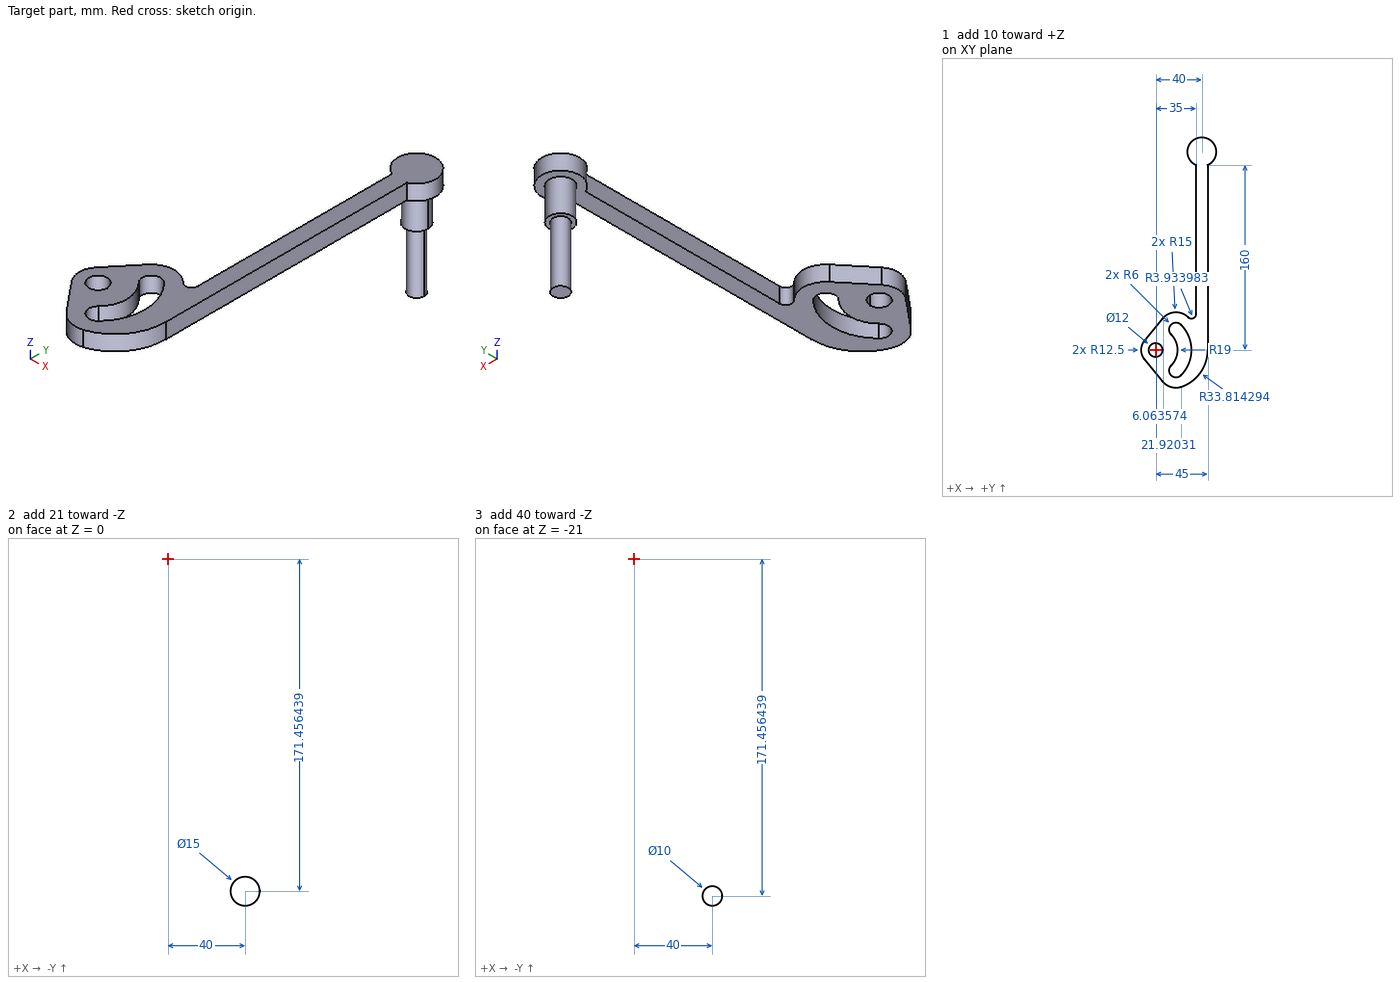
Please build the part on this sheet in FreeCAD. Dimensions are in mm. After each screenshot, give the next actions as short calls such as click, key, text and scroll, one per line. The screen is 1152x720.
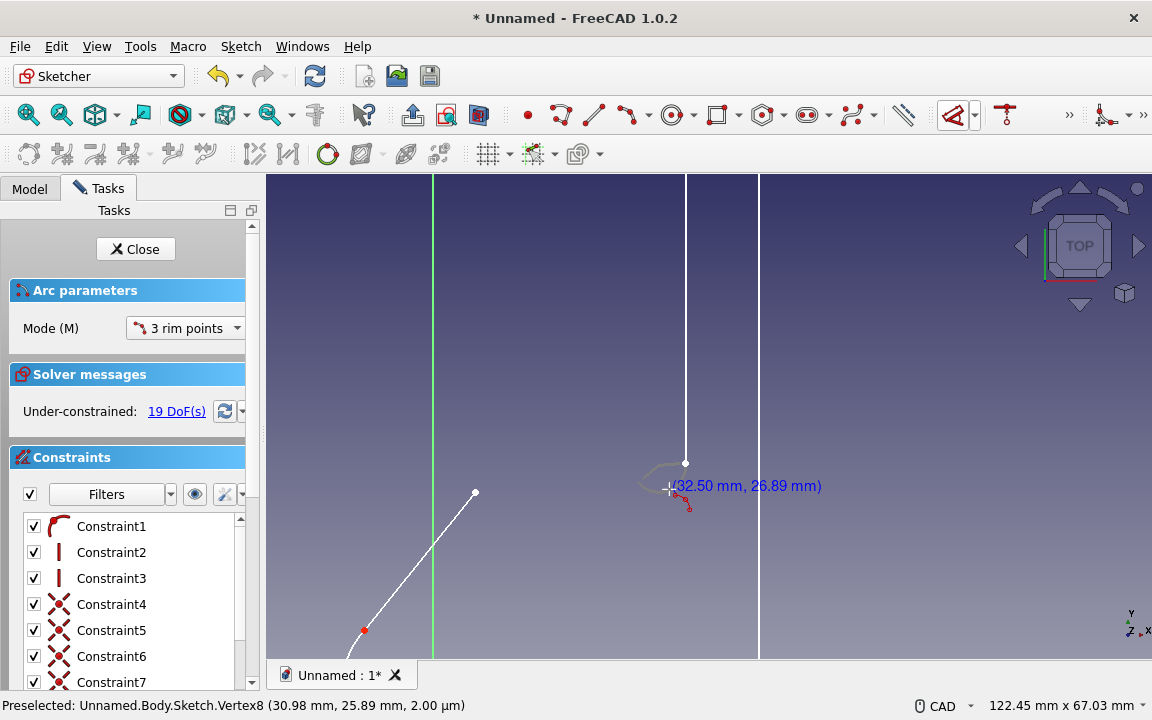
click(669, 487)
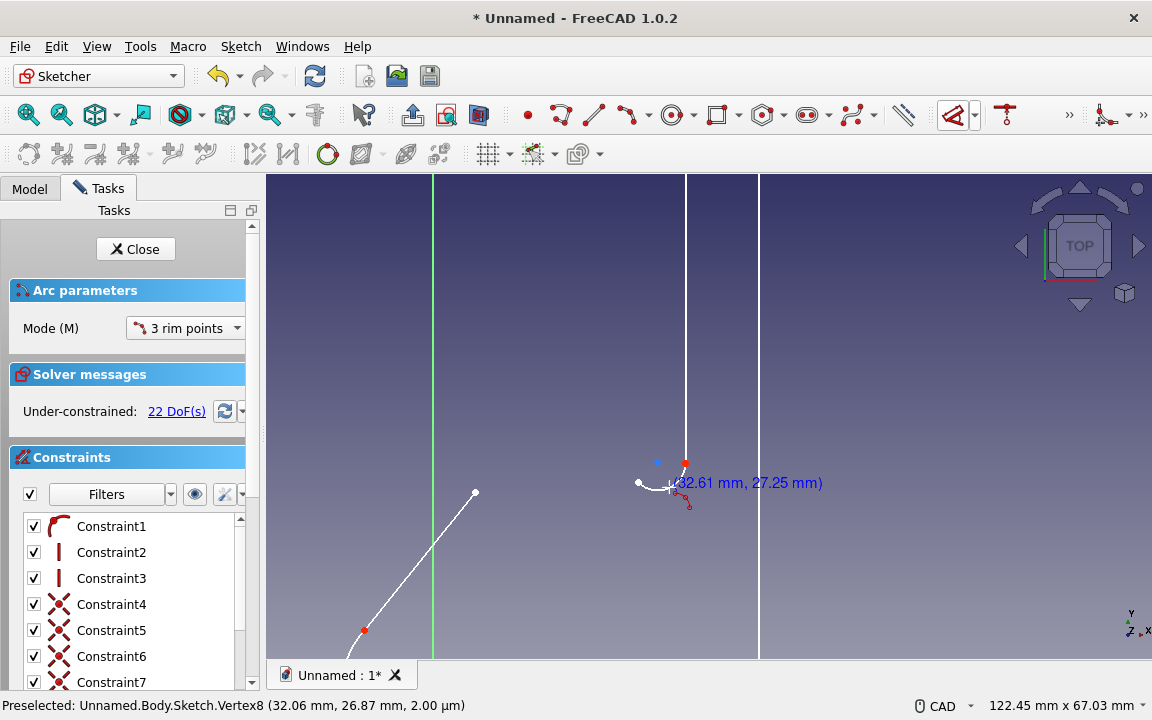
click(638, 482)
click(476, 492)
click(556, 449)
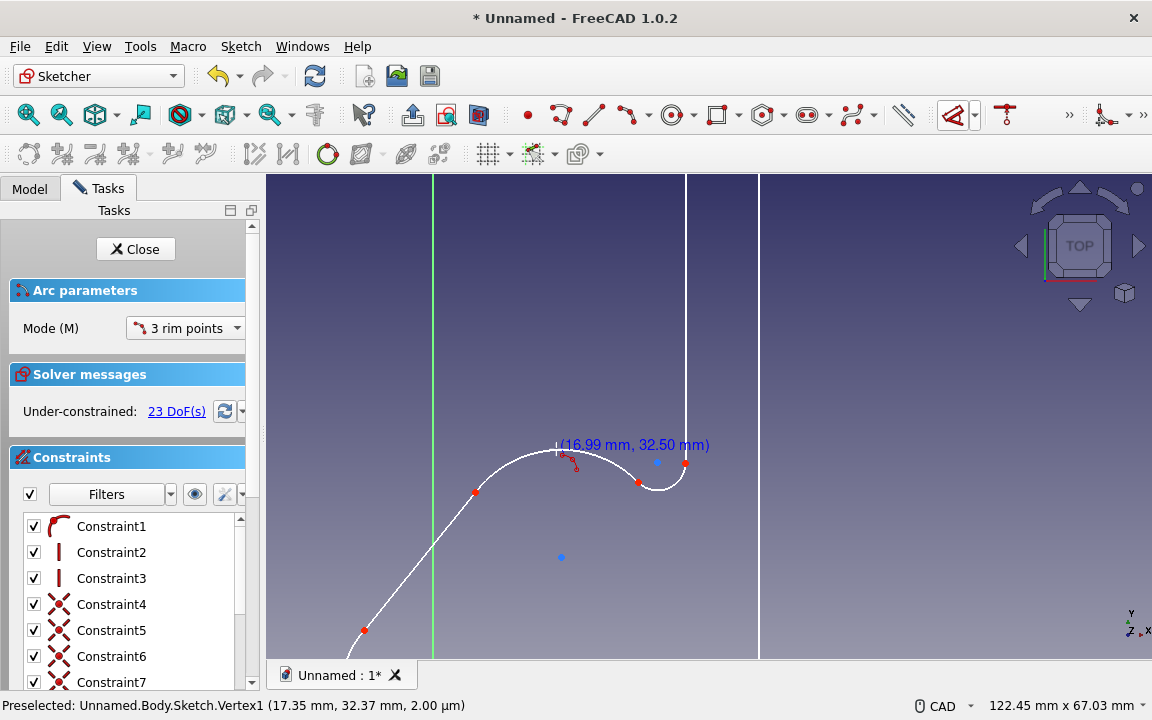
scroll(663, 488, down, 8)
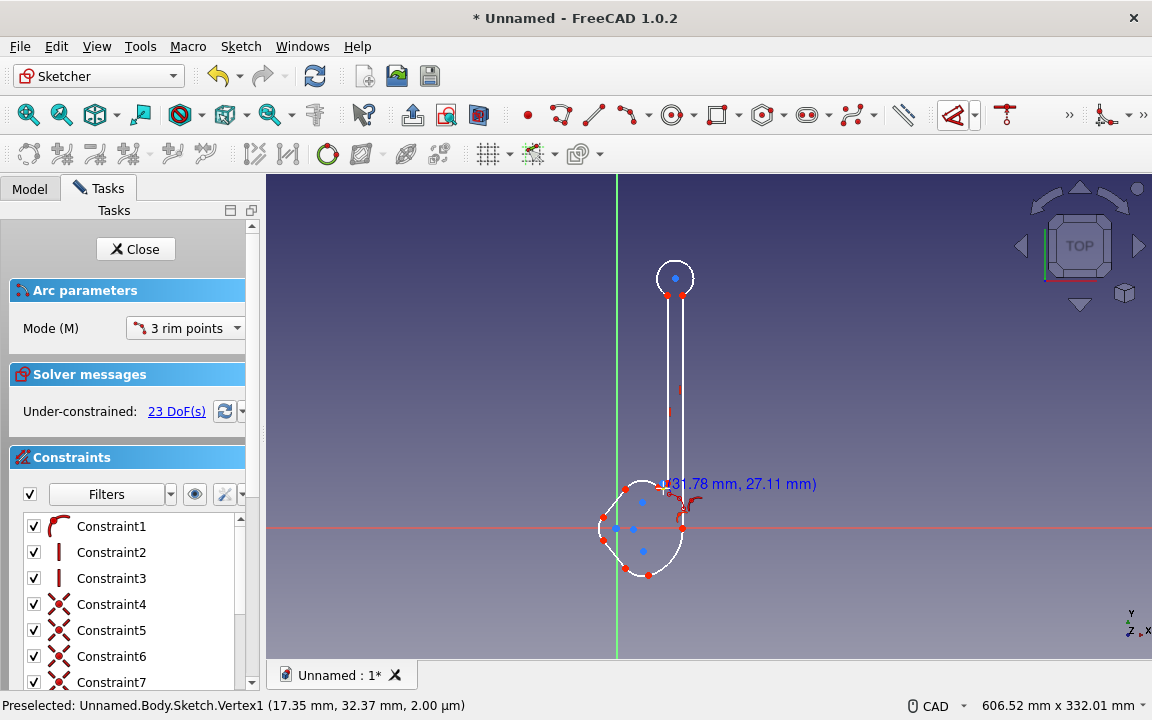
scroll(637, 548, up, 3)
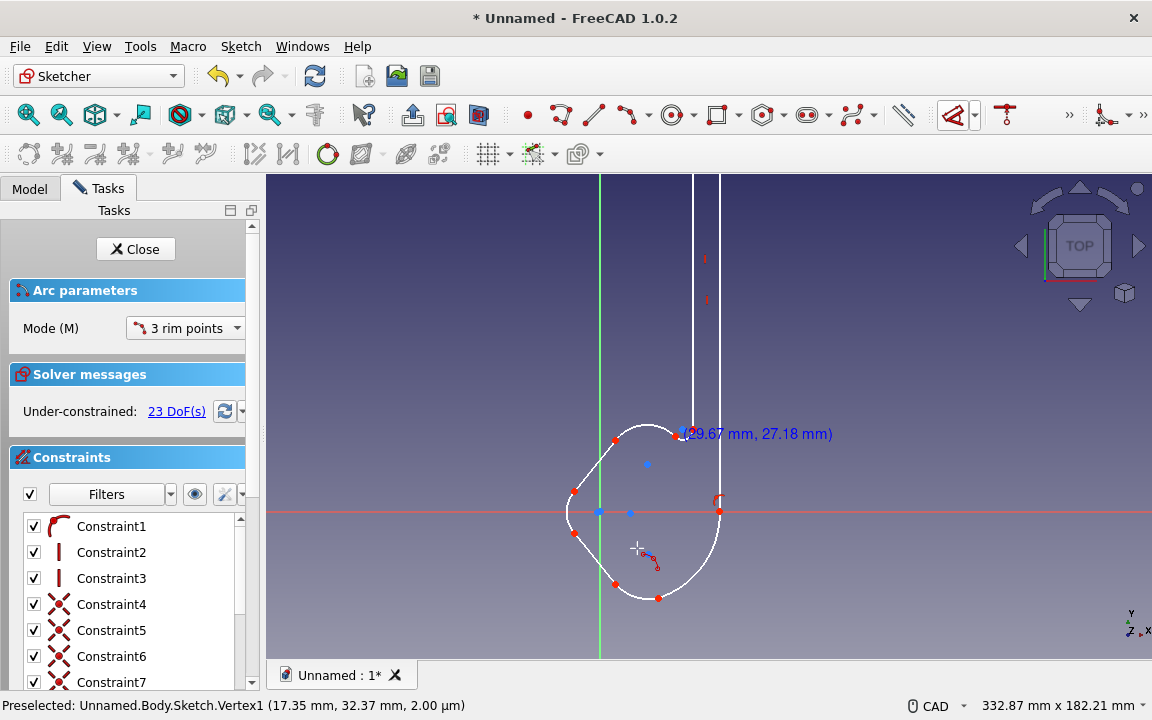
click(636, 547)
click(636, 476)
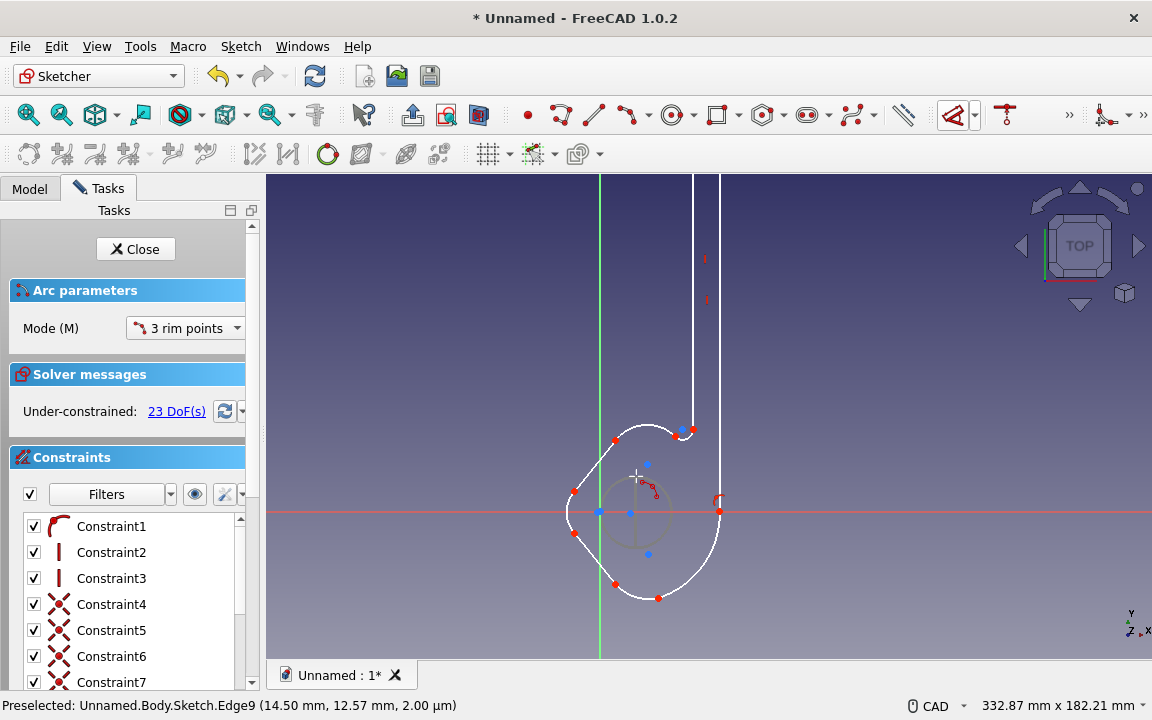
scroll(648, 527, up, 2)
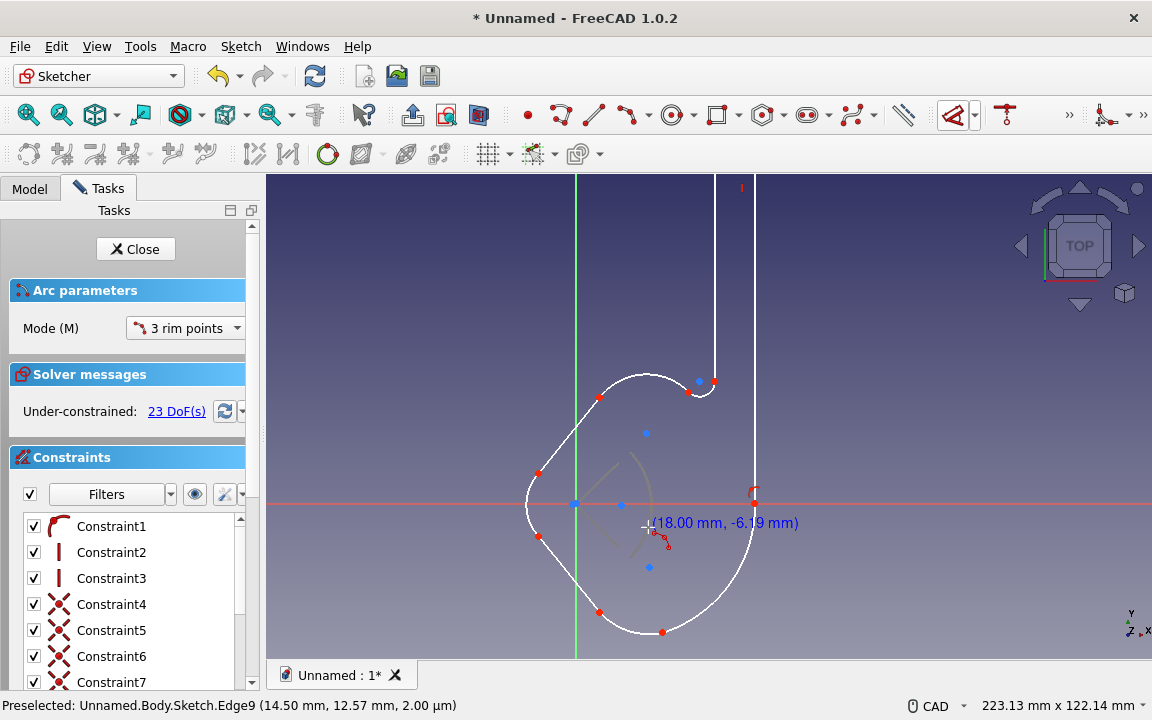
click(648, 527)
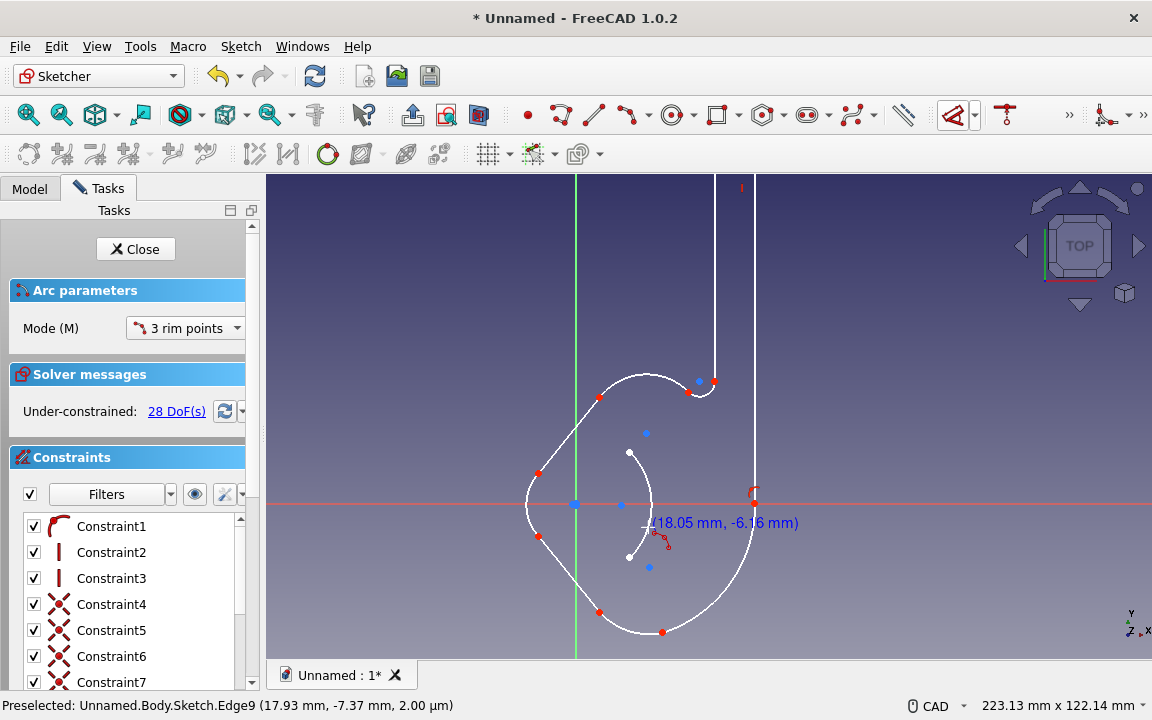
click(630, 452)
click(663, 417)
click(630, 417)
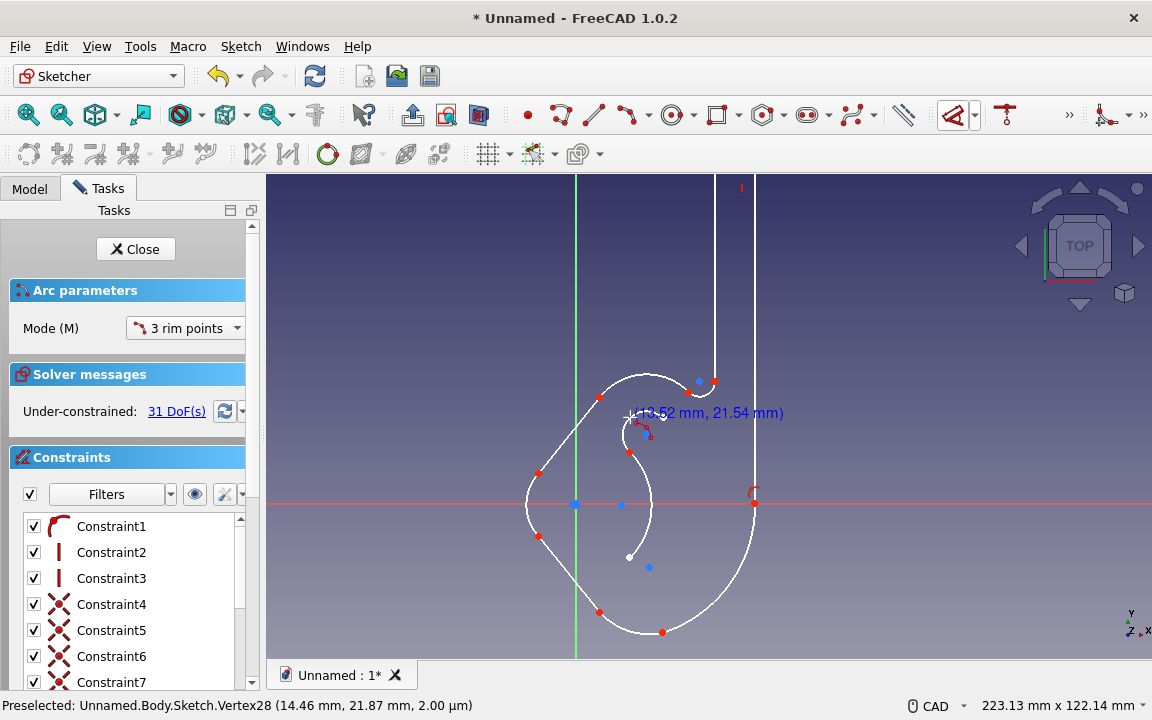
click(663, 418)
click(663, 591)
click(693, 542)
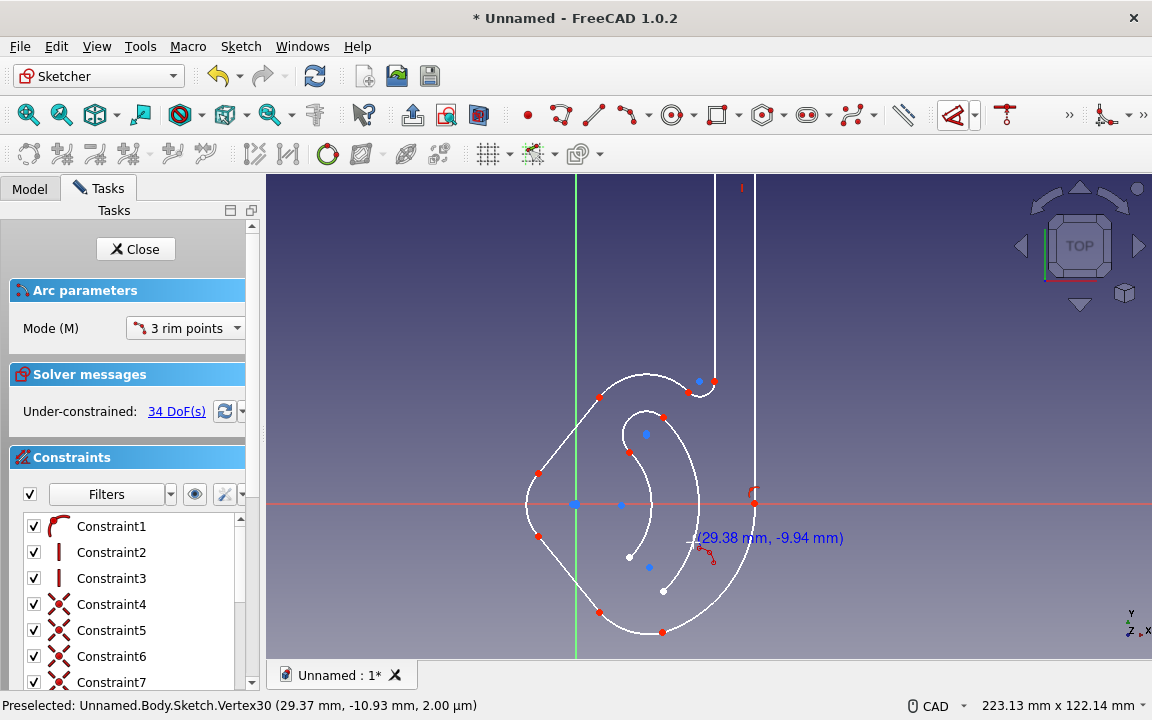
click(663, 592)
click(630, 558)
click(630, 591)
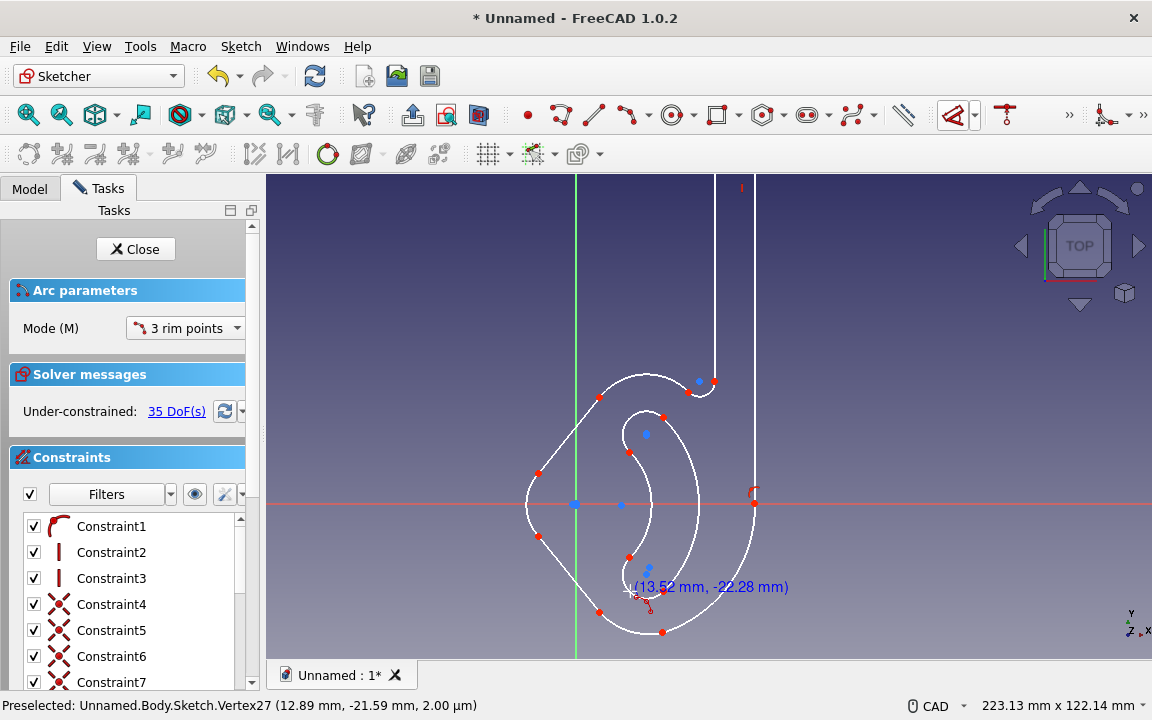
key(g)
key(c)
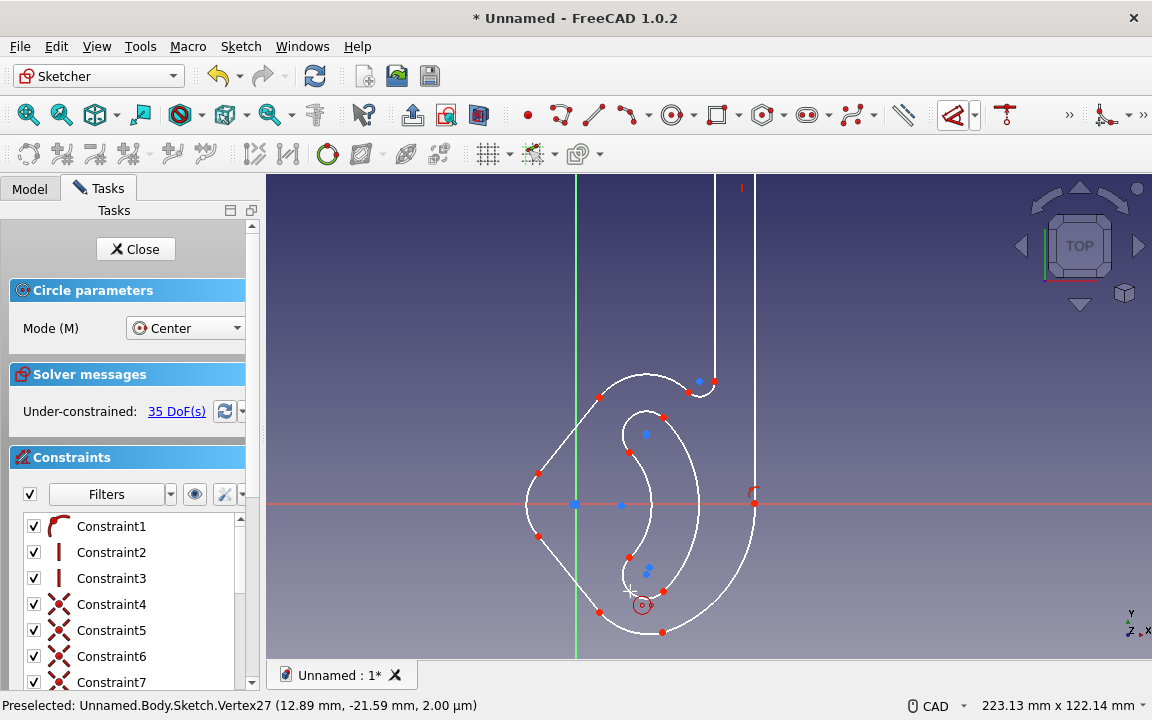
click(576, 504)
click(593, 487)
key(Escape)